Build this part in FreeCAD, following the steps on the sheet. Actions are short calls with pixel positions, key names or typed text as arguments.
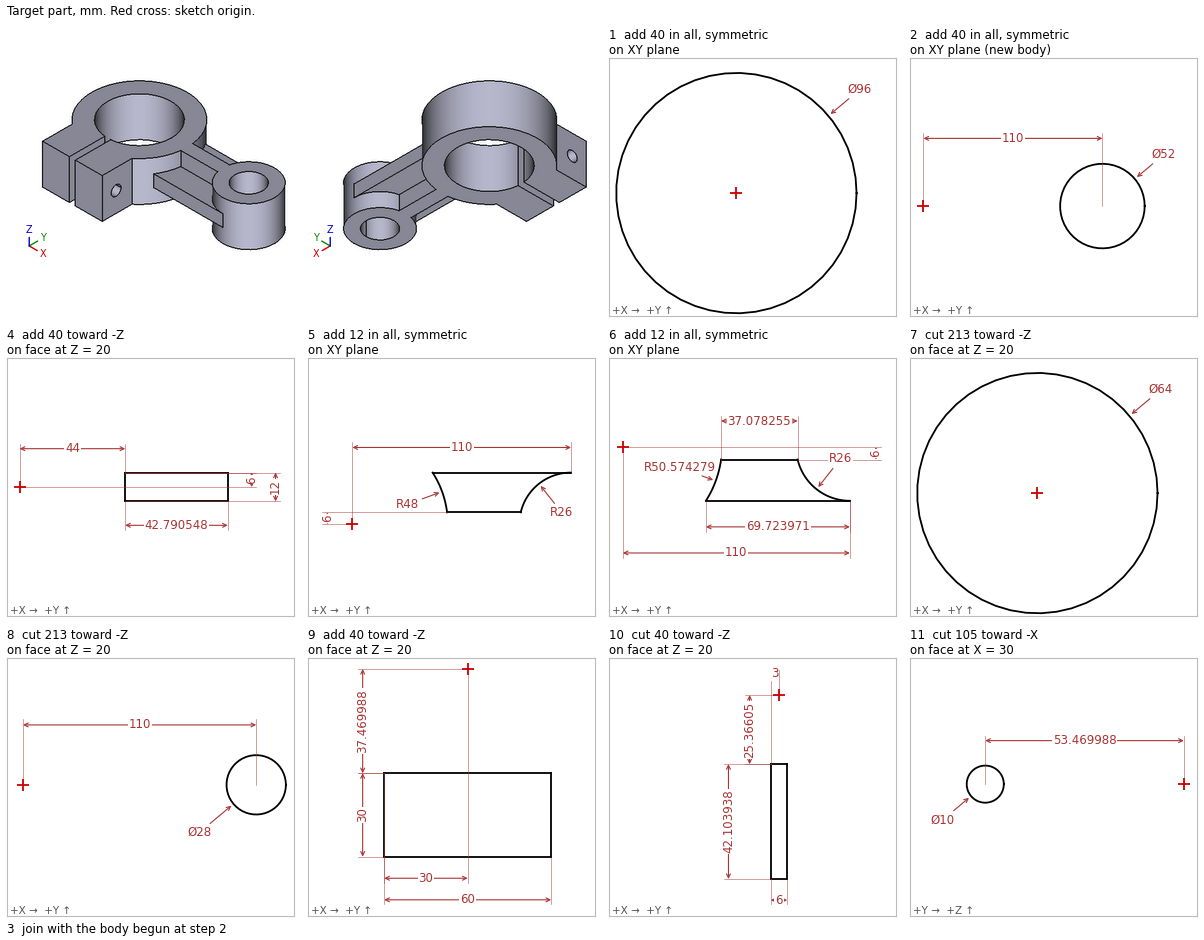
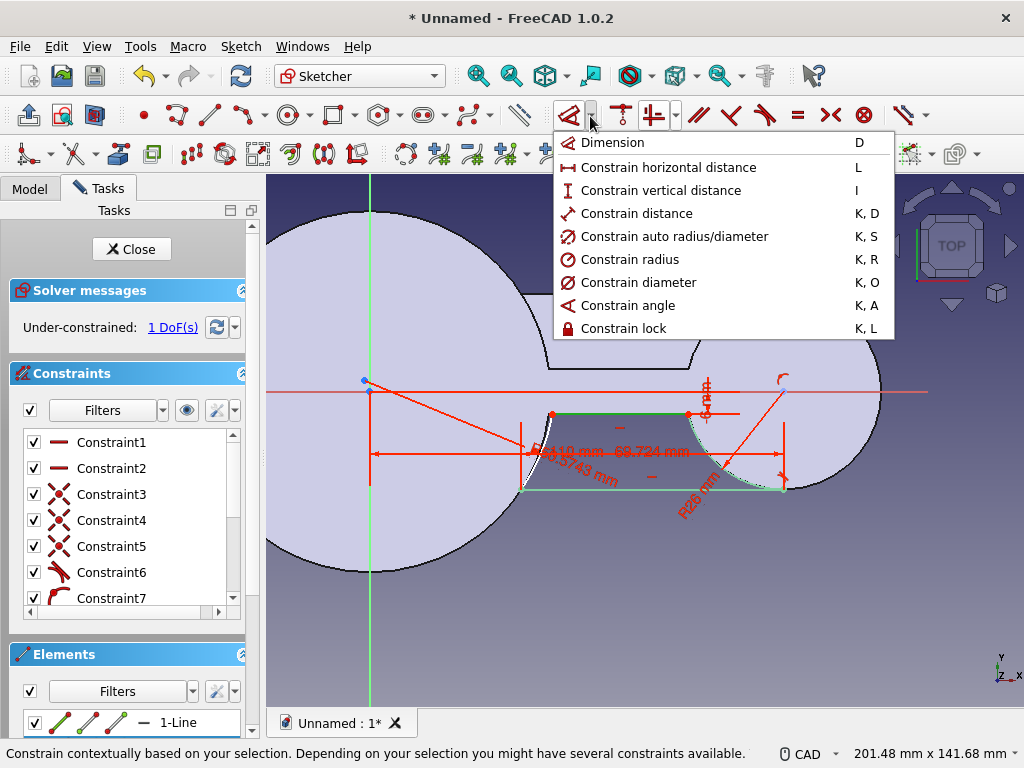
click(724, 168)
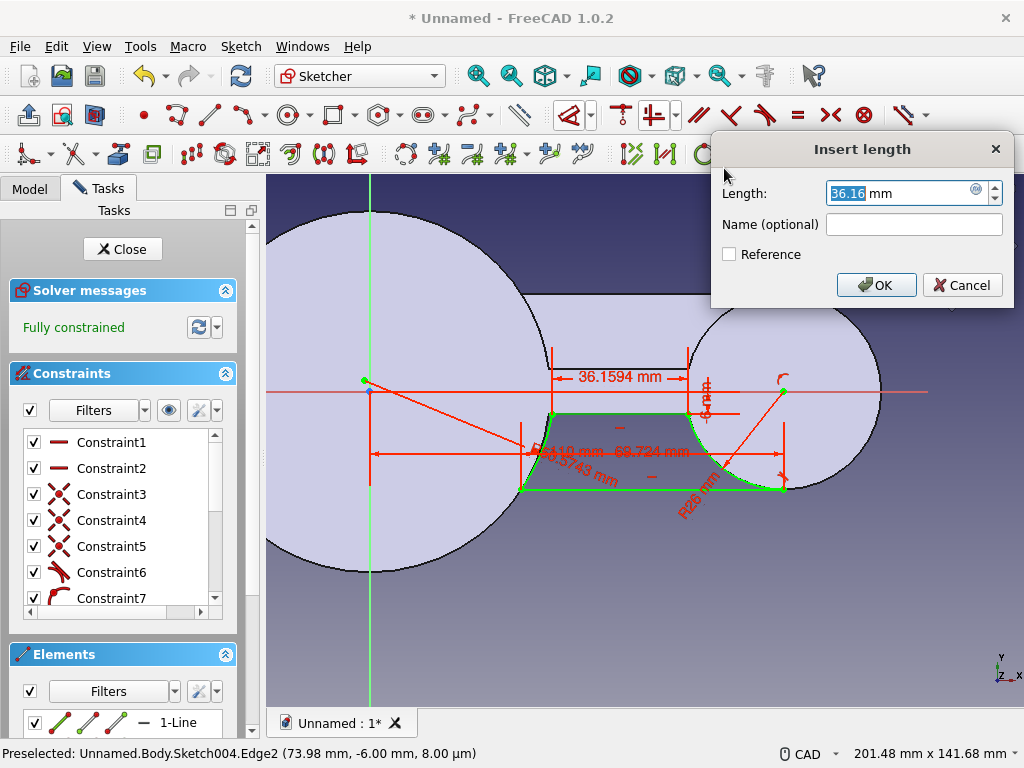
text(37.078255)
key(Return)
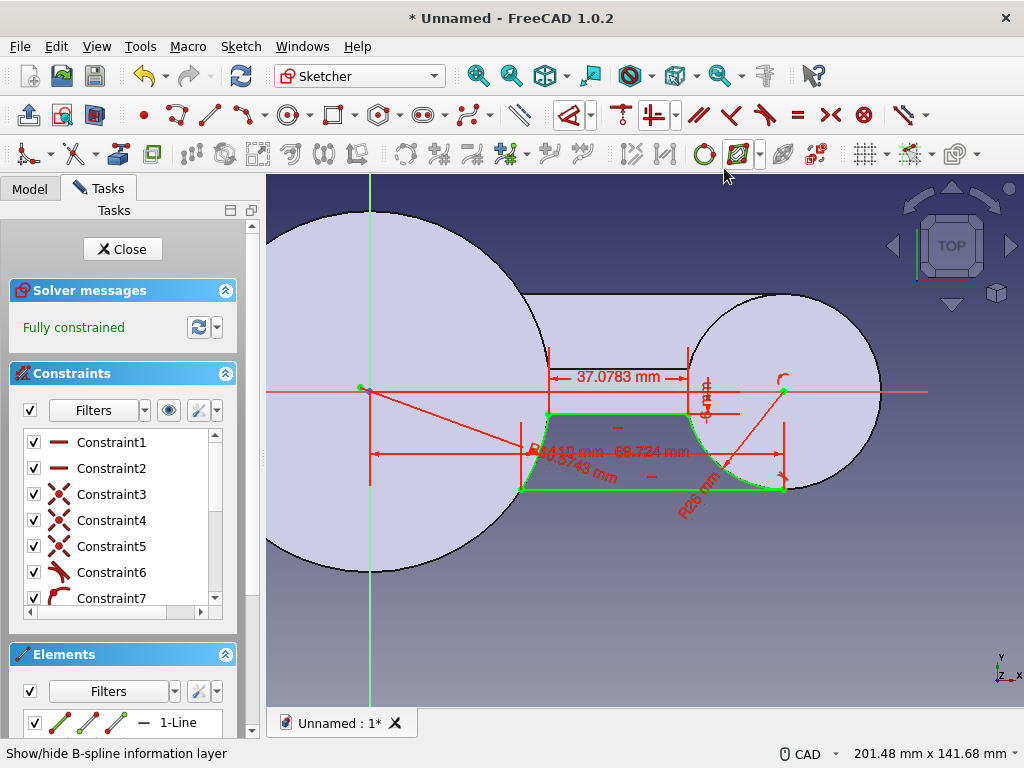
click(123, 249)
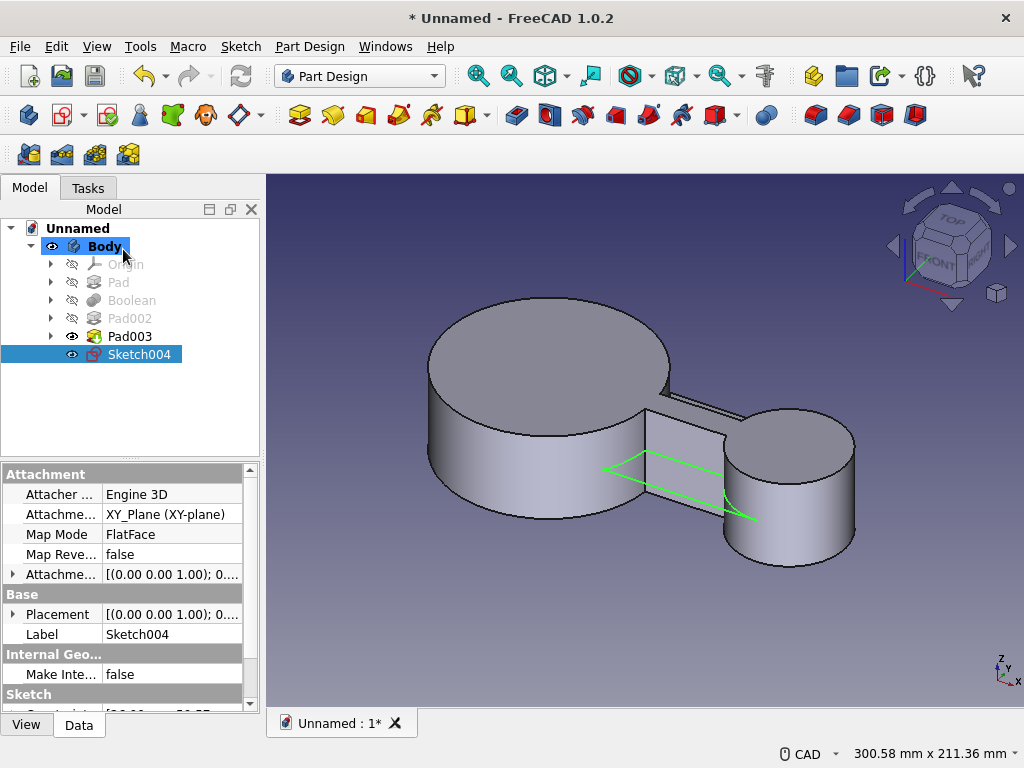
click(300, 116)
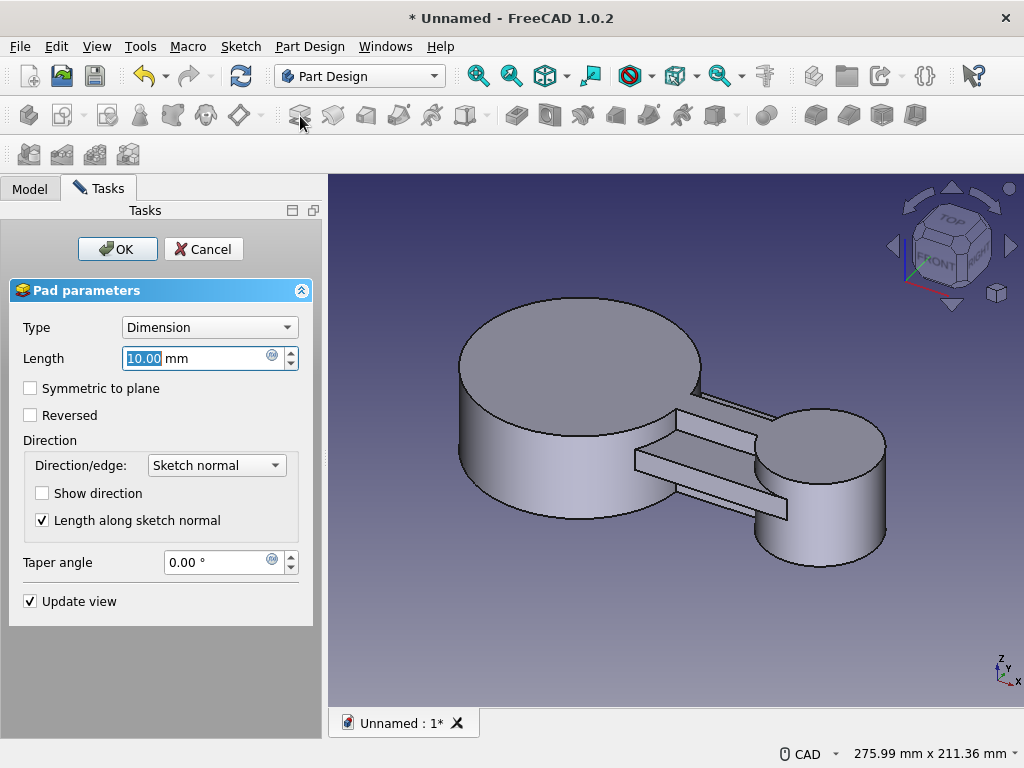
text(12)
key(Tab)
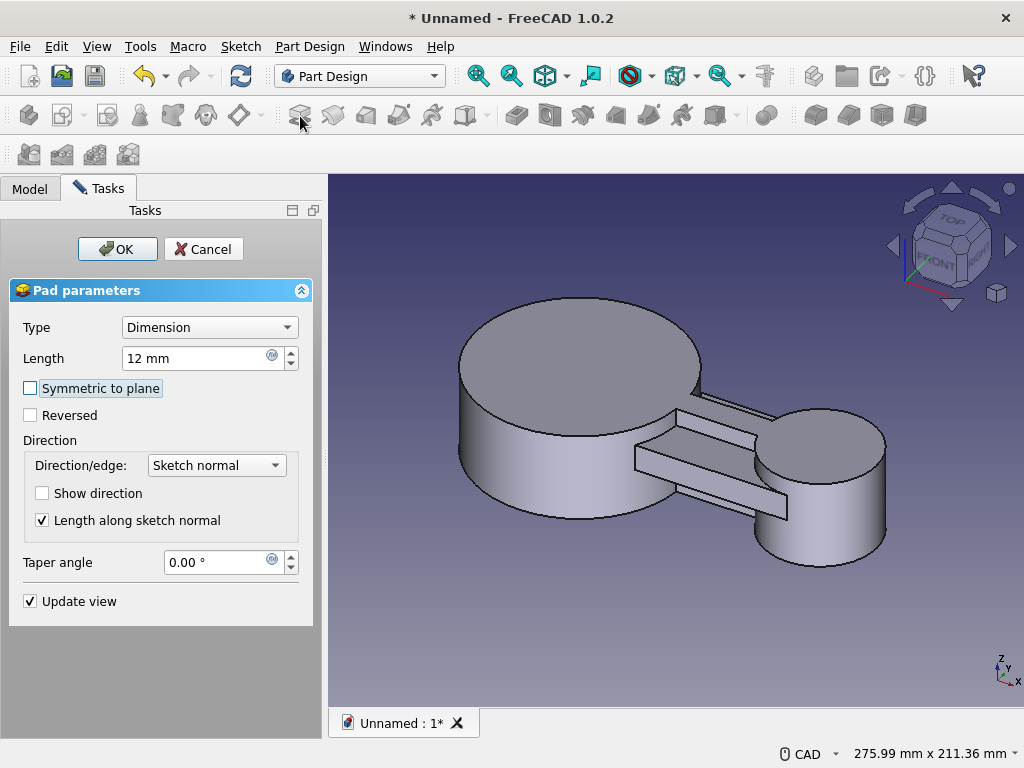
click(31, 388)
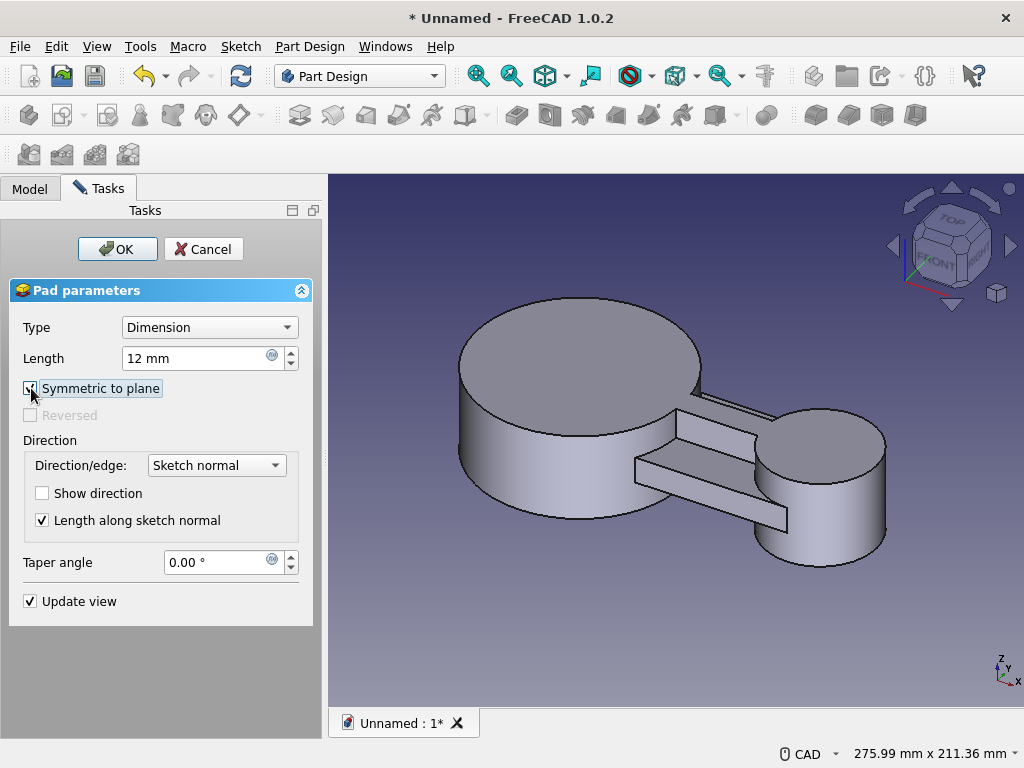
click(118, 249)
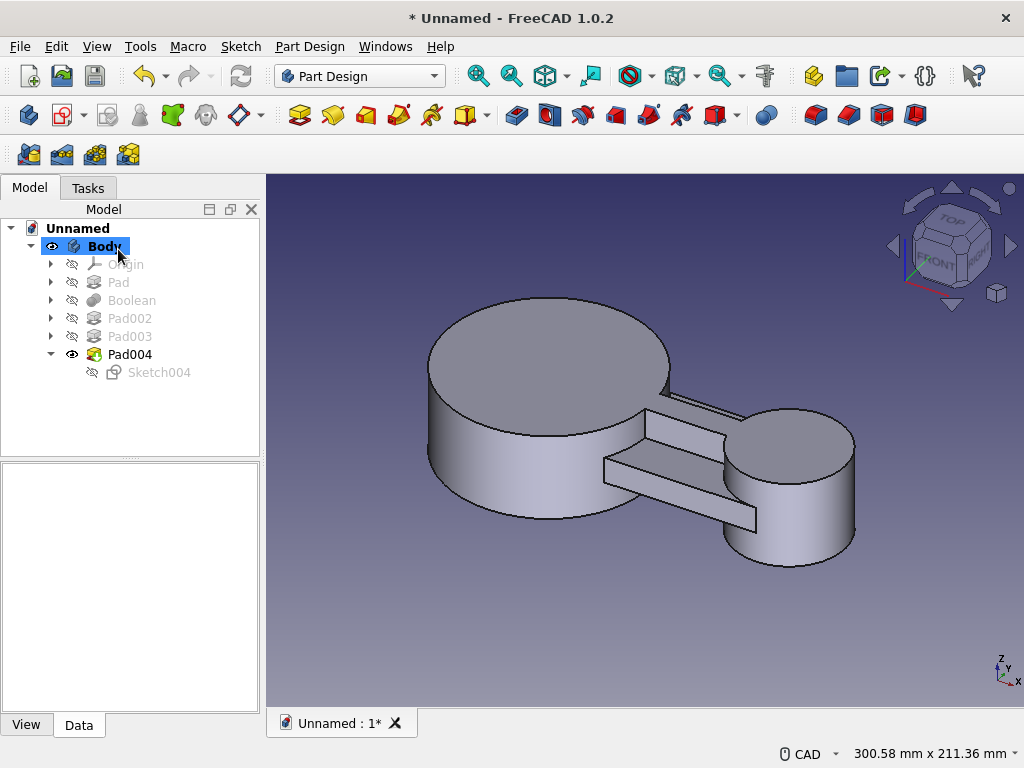
click(530, 360)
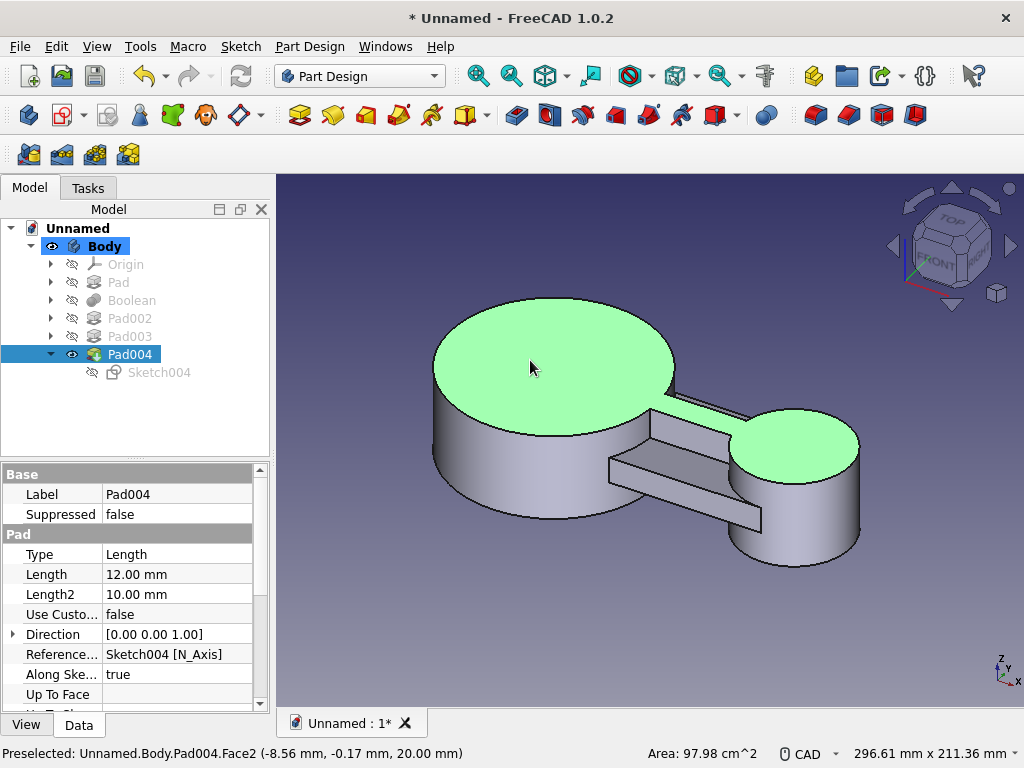
click(62, 116)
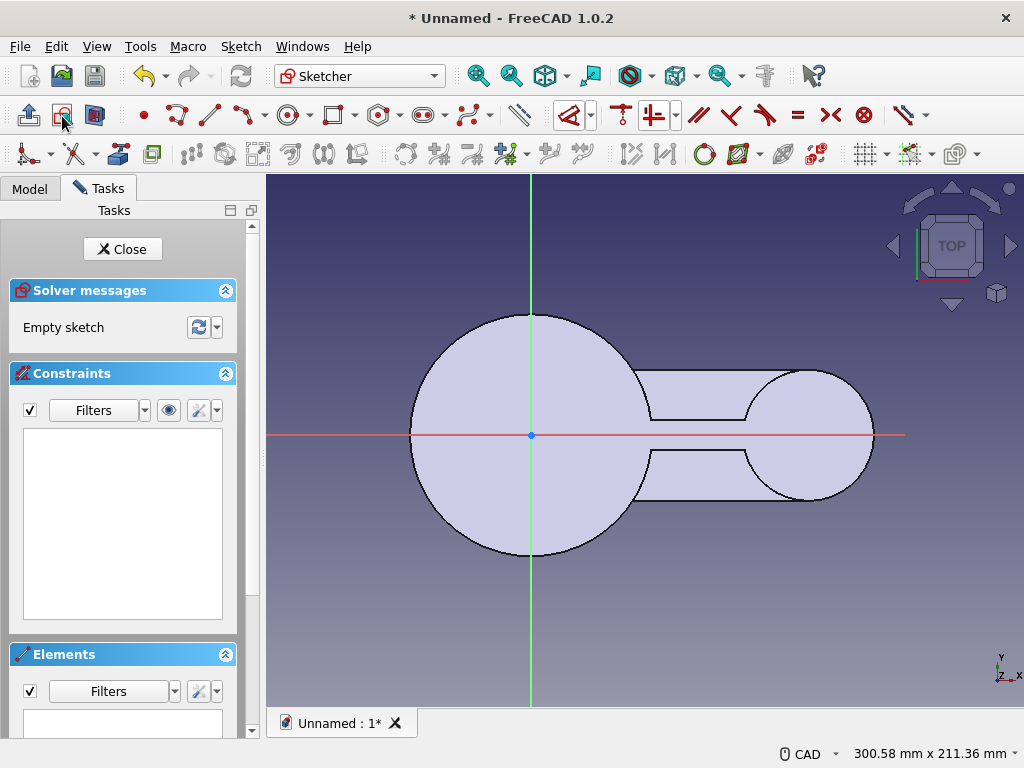
scroll(494, 431, up, 4)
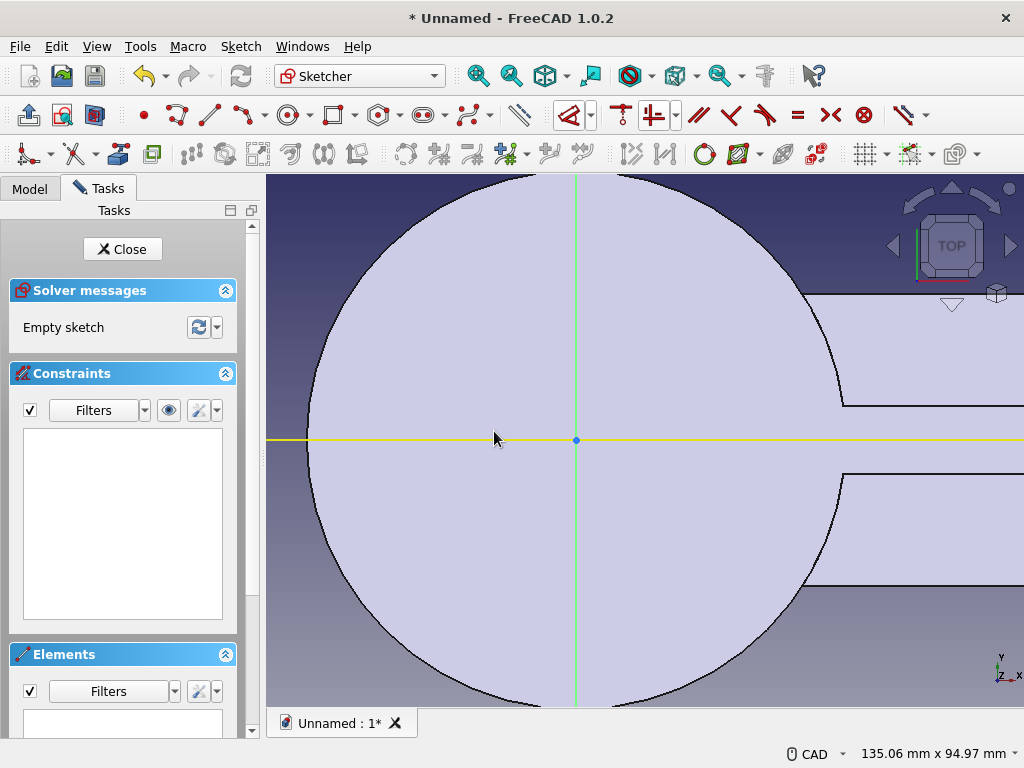
click(288, 116)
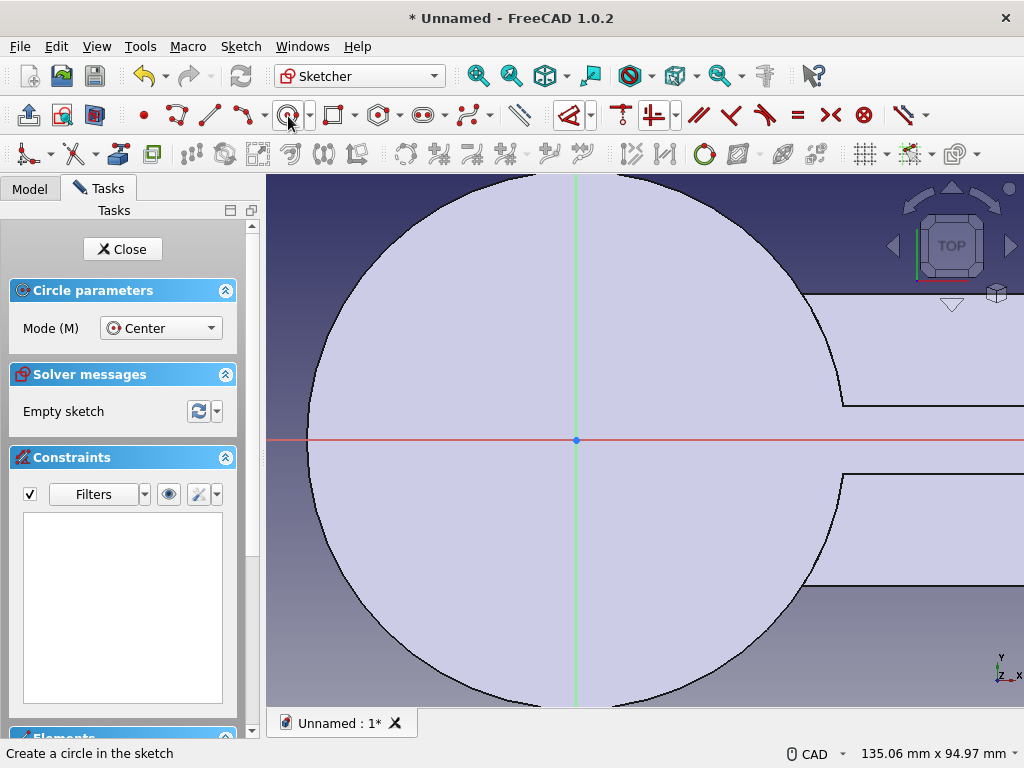
click(576, 440)
click(703, 313)
key(Escape)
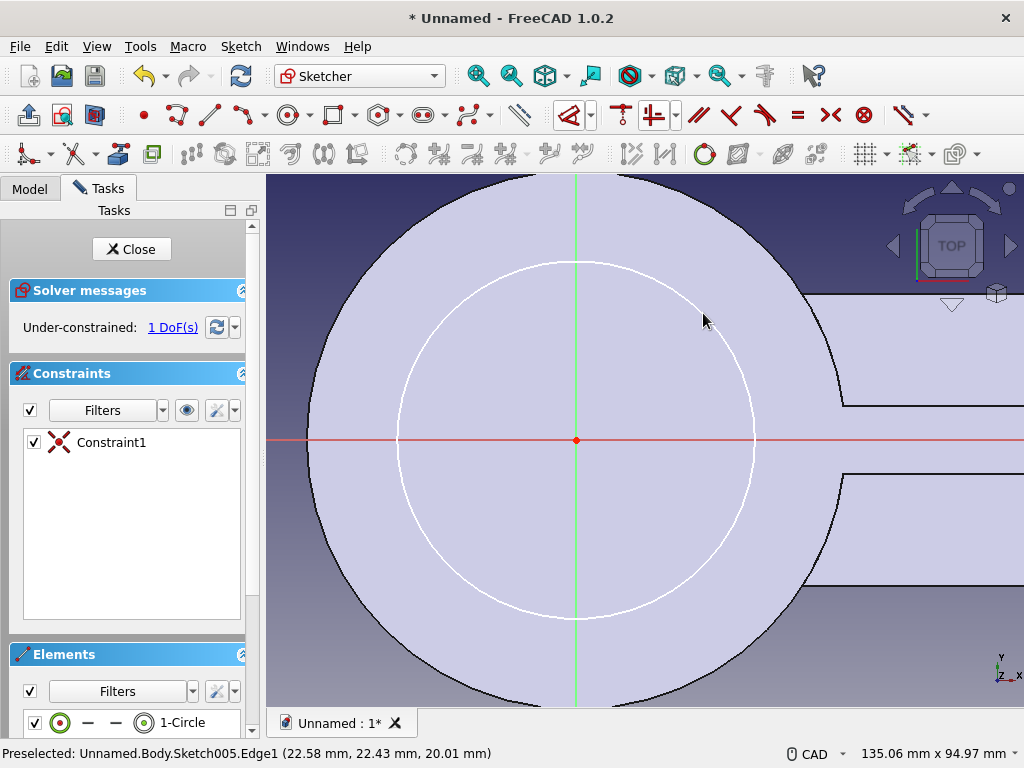
click(702, 313)